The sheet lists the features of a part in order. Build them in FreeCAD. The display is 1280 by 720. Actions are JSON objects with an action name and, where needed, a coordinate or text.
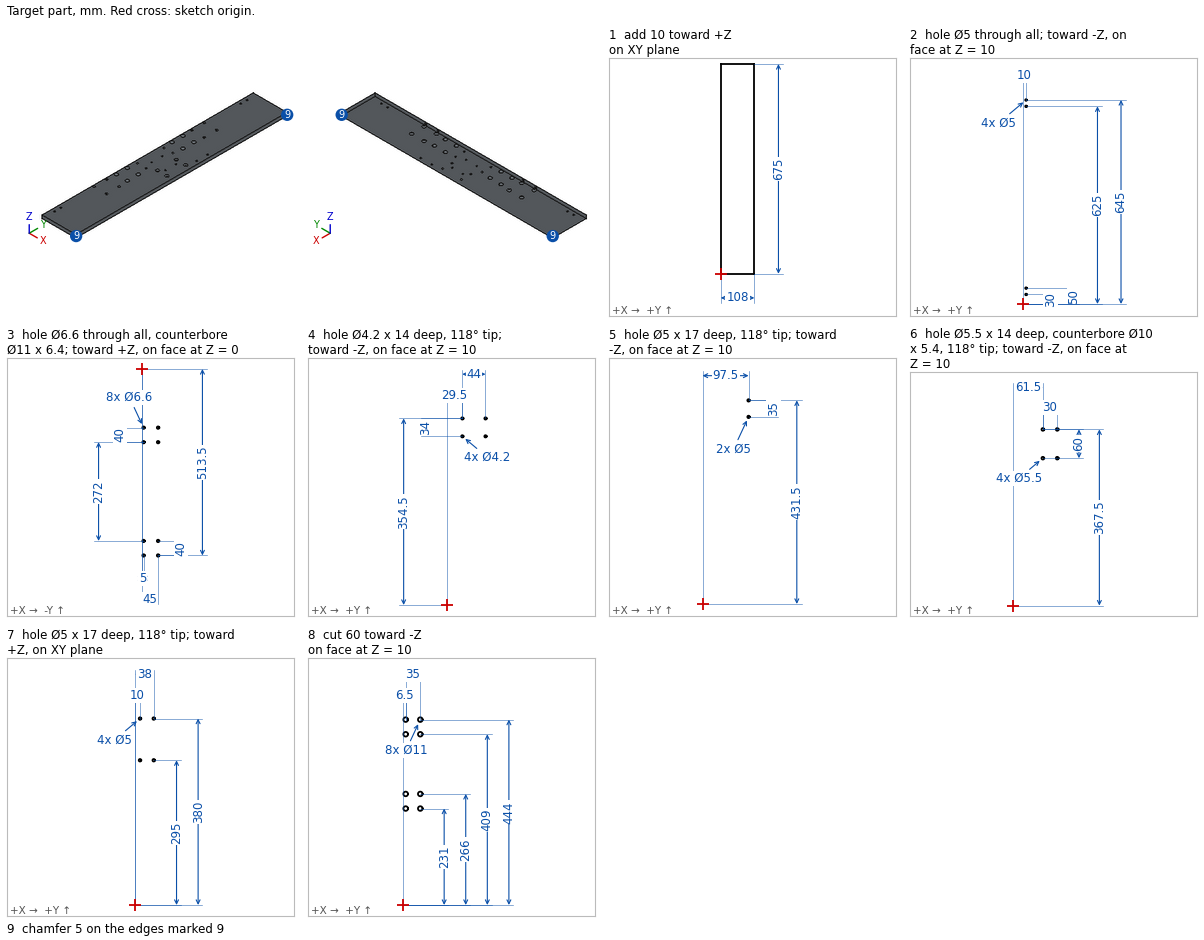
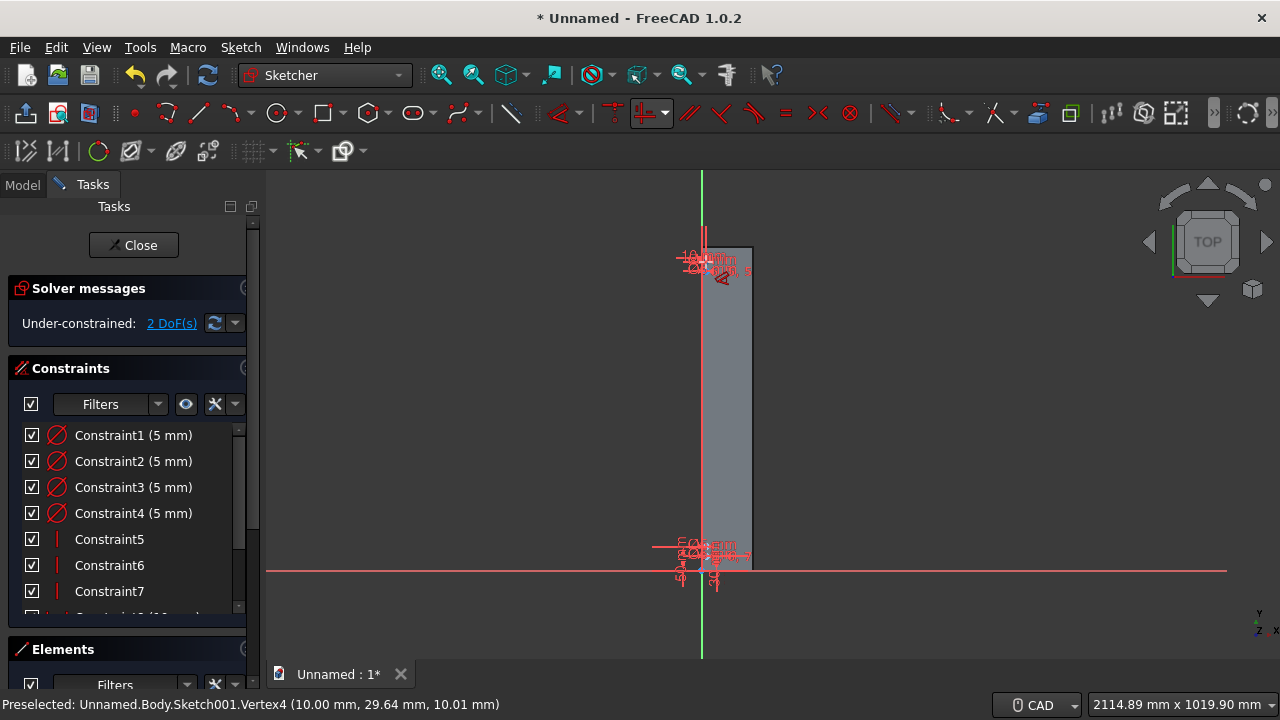
{"action": "left_click", "coordinate": [706, 261]}
{"action": "left_click", "coordinate": [665, 446]}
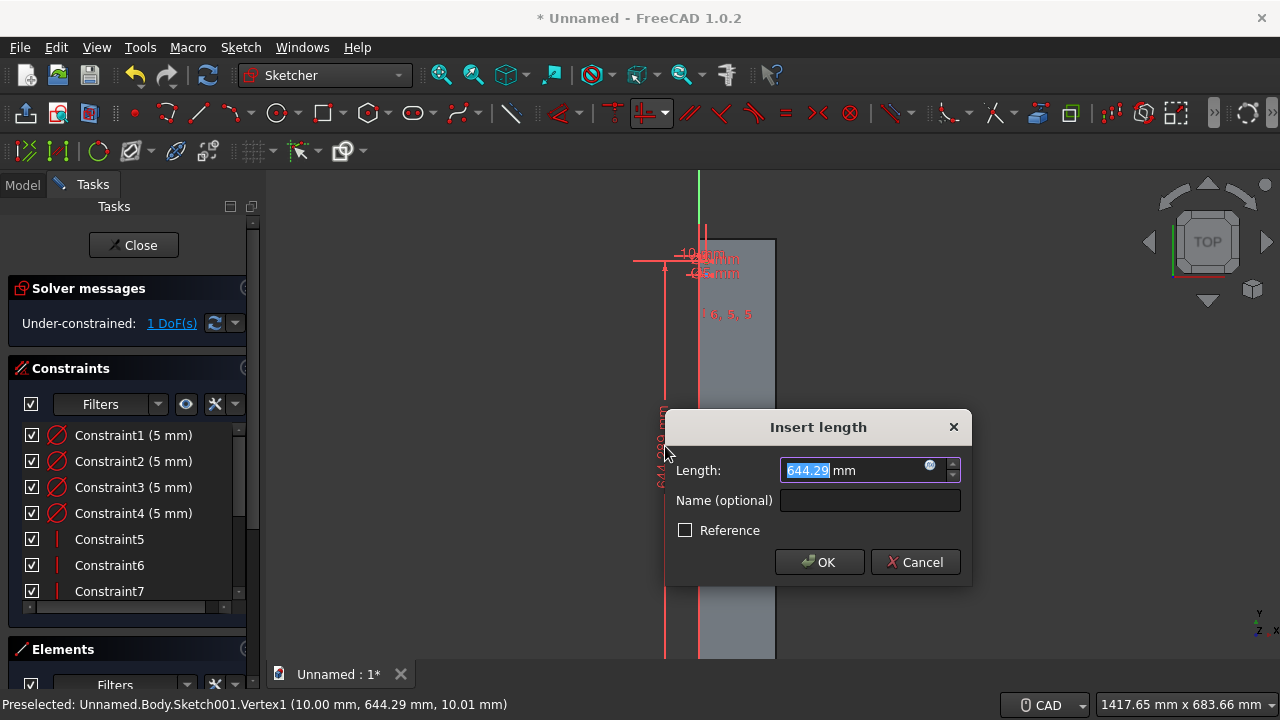
{"action": "type", "text": "645"}
{"action": "key", "text": "Return"}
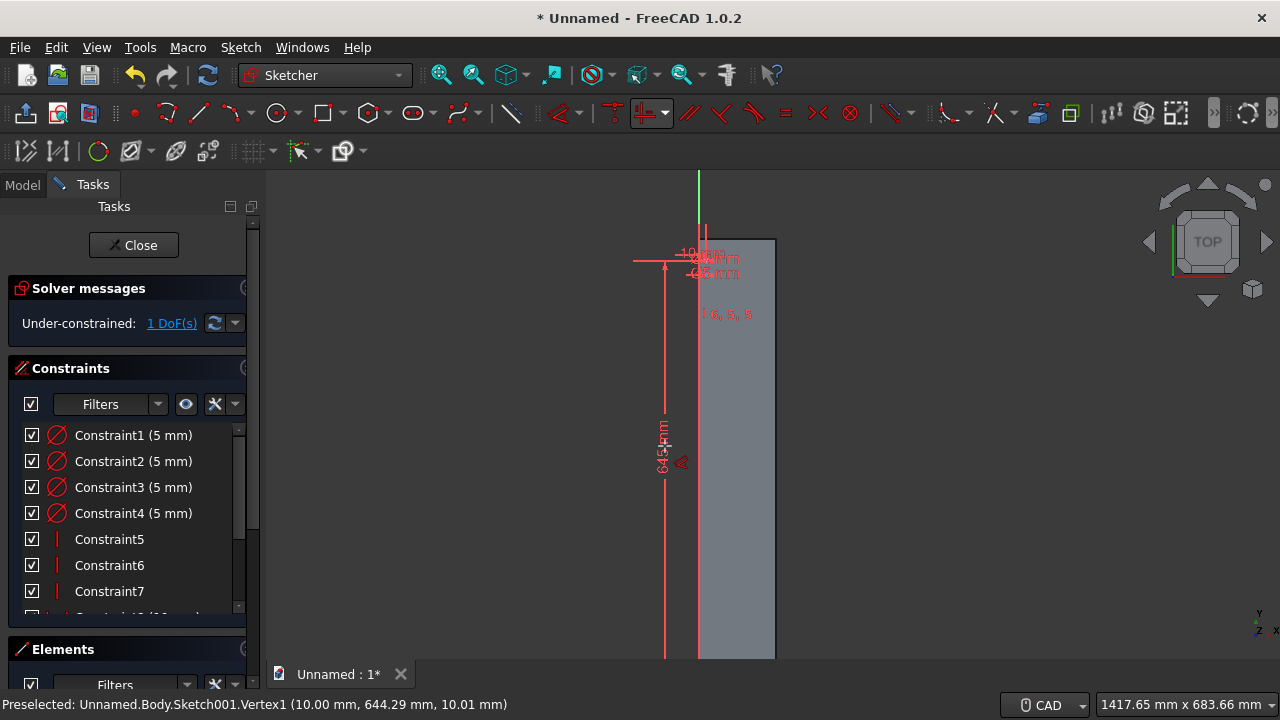
{"action": "left_click", "coordinate": [706, 275]}
{"action": "left_click", "coordinate": [665, 371]}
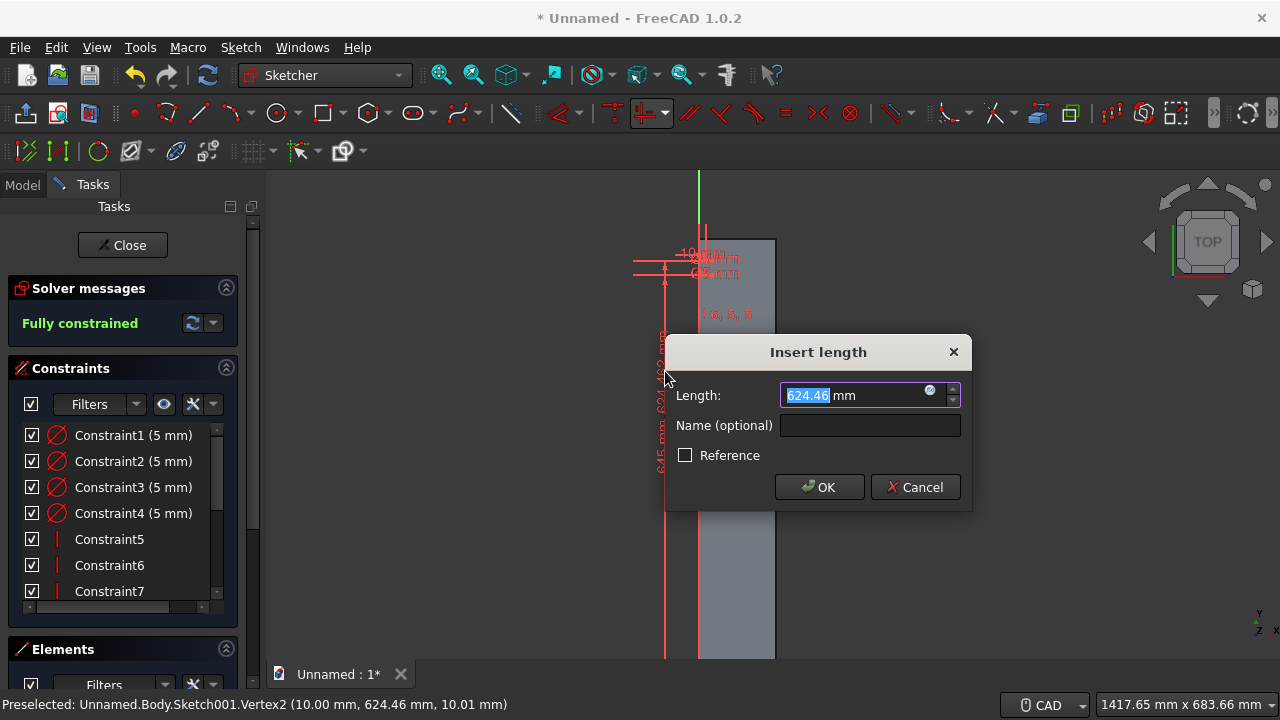
{"action": "type", "text": "625"}
{"action": "key", "text": "Return"}
{"action": "key", "text": "Escape"}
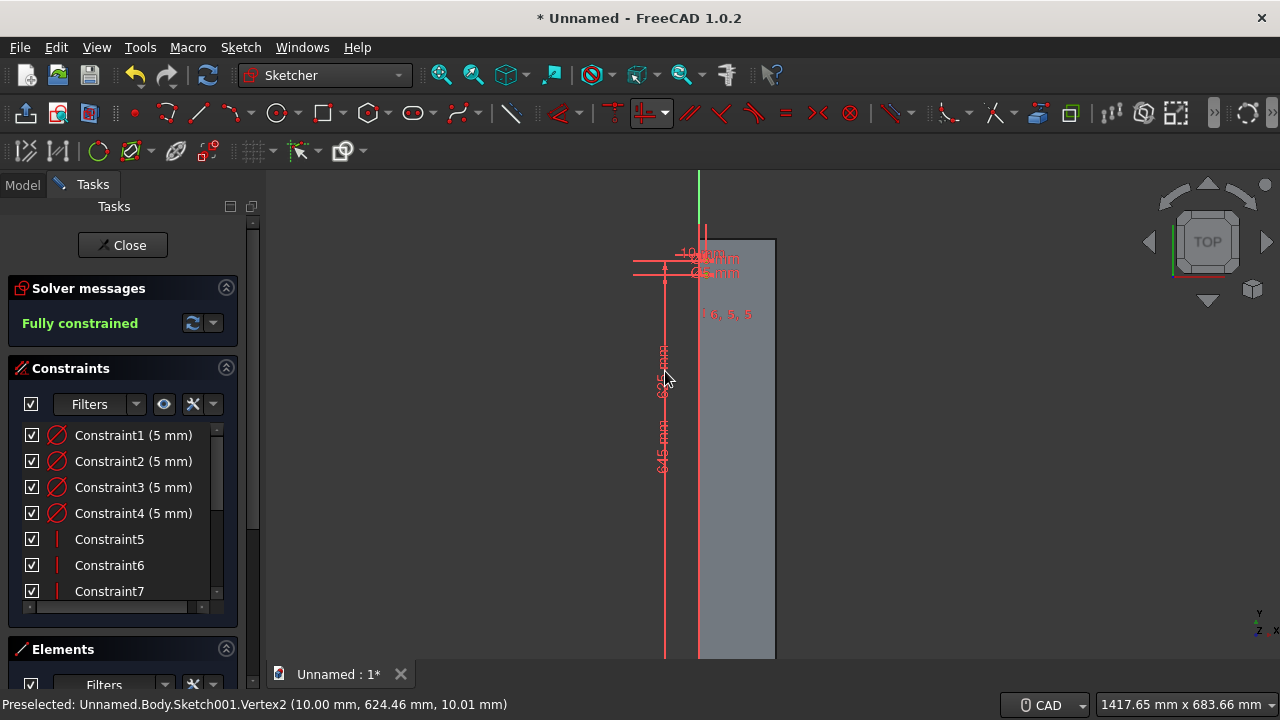
{"action": "left_click", "coordinate": [123, 245]}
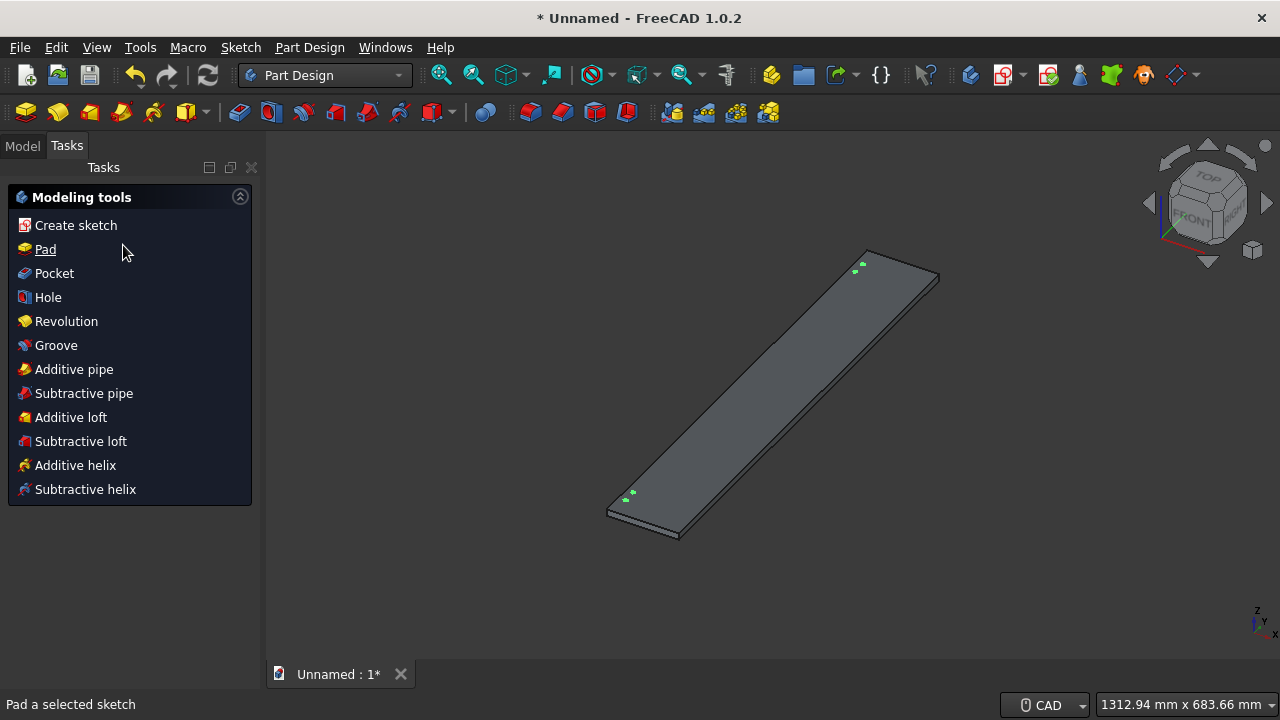
{"action": "left_click", "coordinate": [272, 112]}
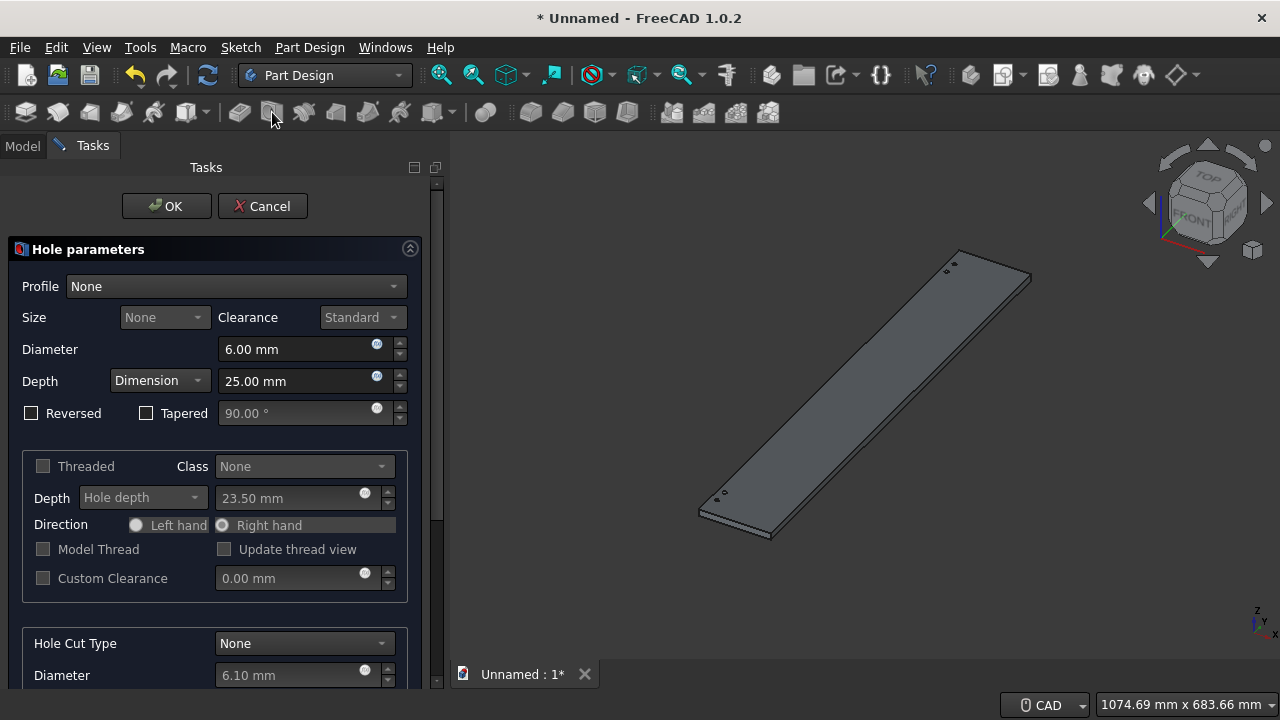
{"action": "triple_click", "coordinate": [305, 349]}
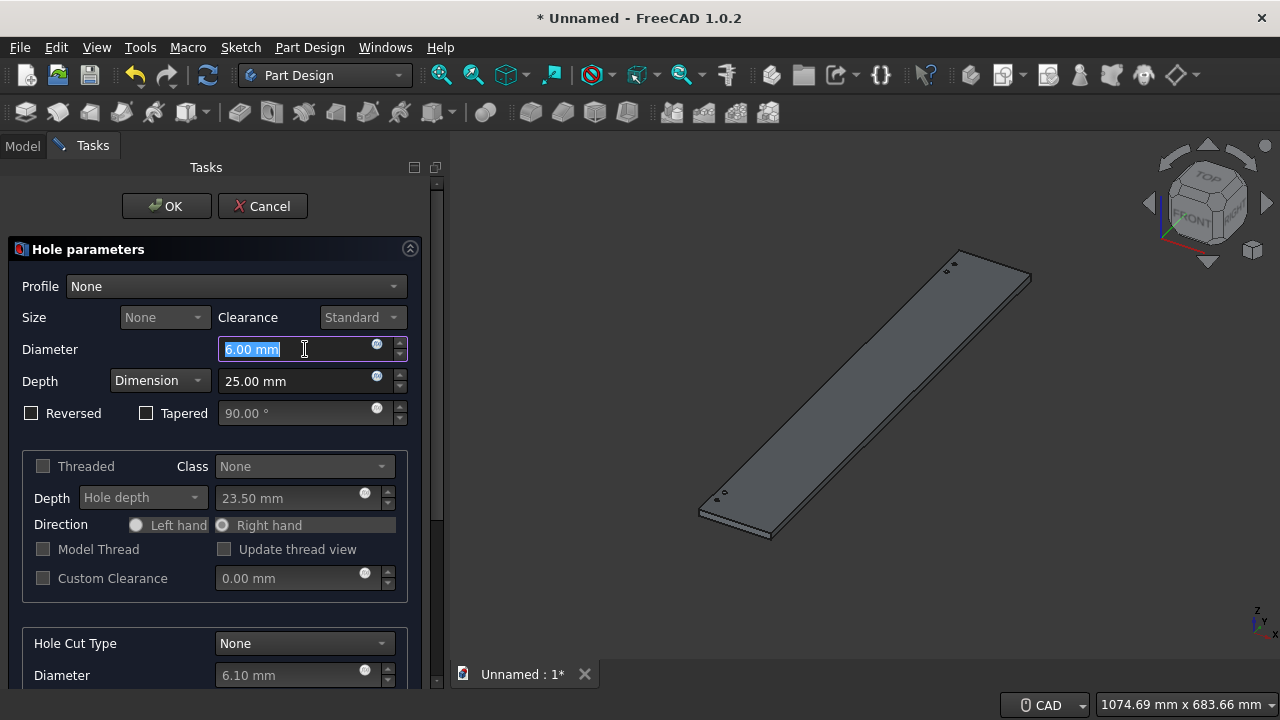
{"action": "type", "text": "5"}
{"action": "key", "text": "Tab"}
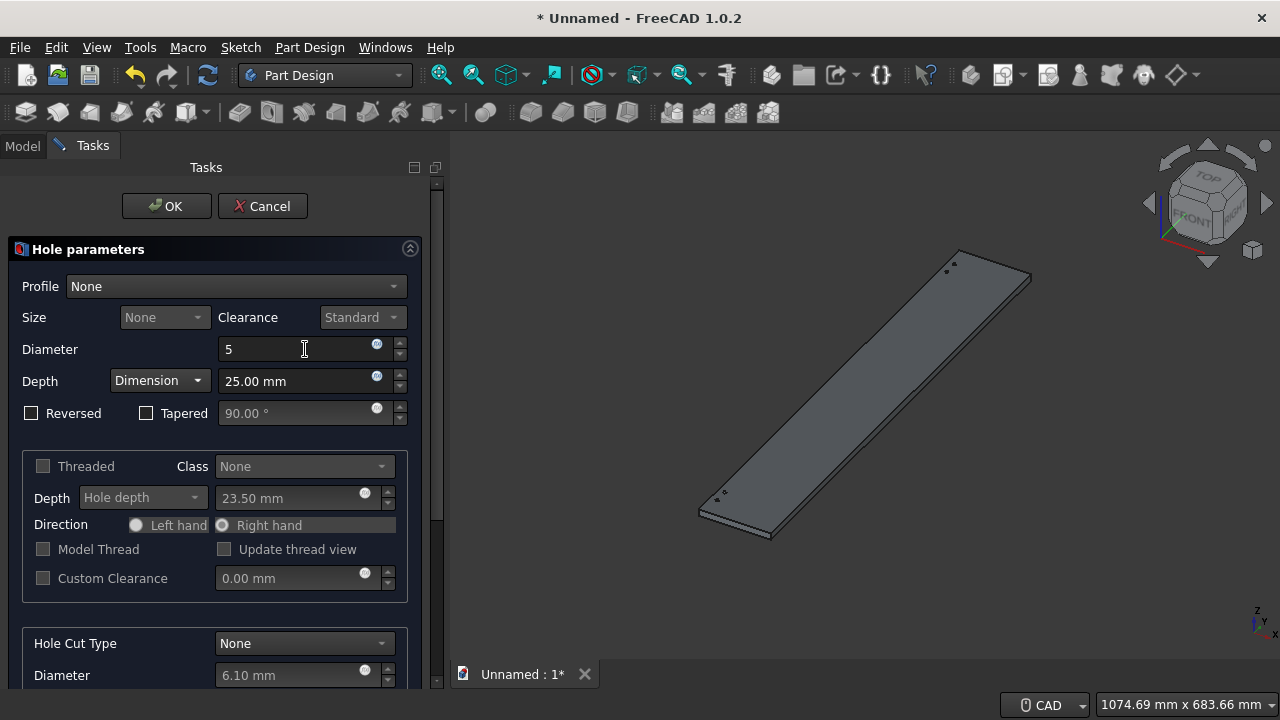
{"action": "left_click", "coordinate": [161, 380]}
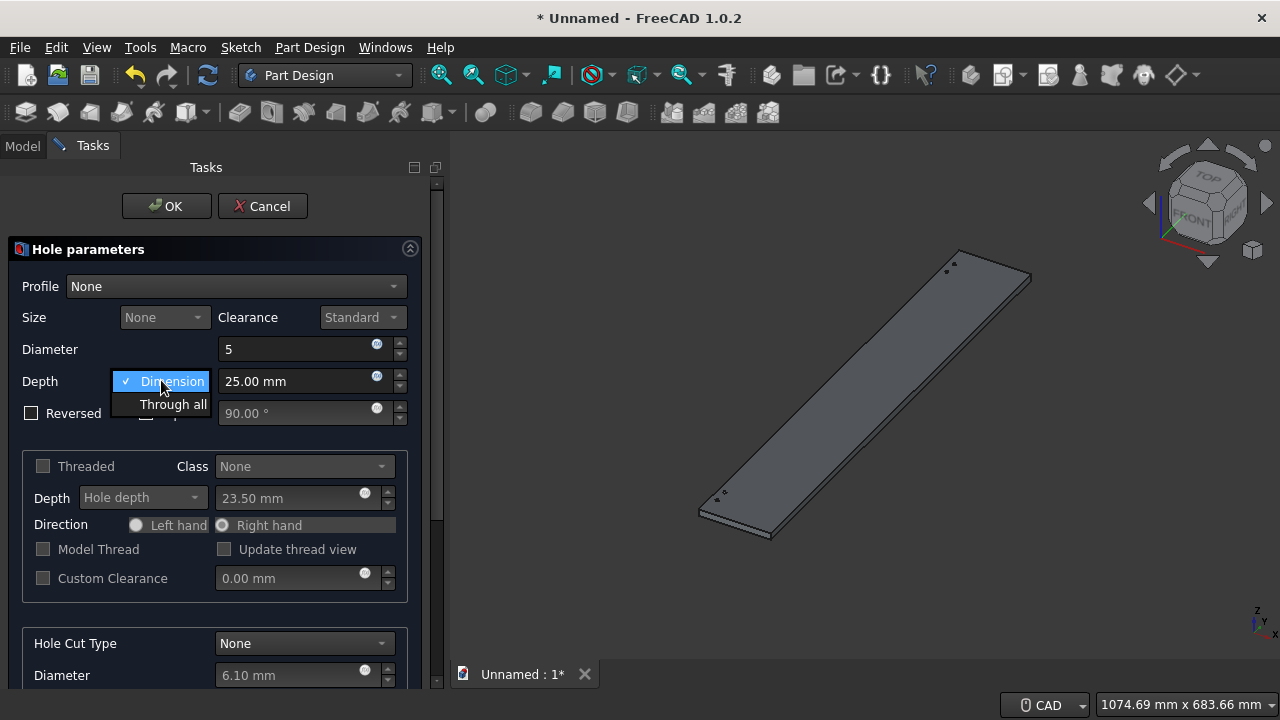
{"action": "left_click", "coordinate": [160, 404]}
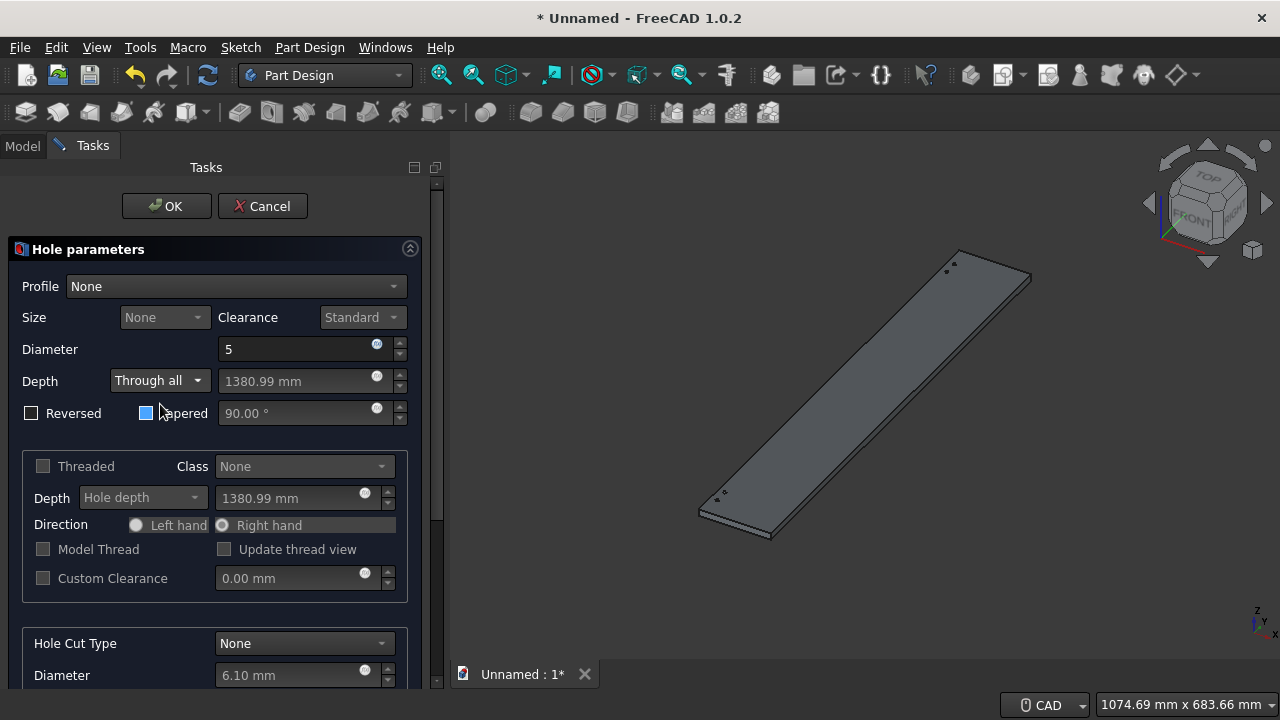
{"action": "left_click", "coordinate": [167, 206]}